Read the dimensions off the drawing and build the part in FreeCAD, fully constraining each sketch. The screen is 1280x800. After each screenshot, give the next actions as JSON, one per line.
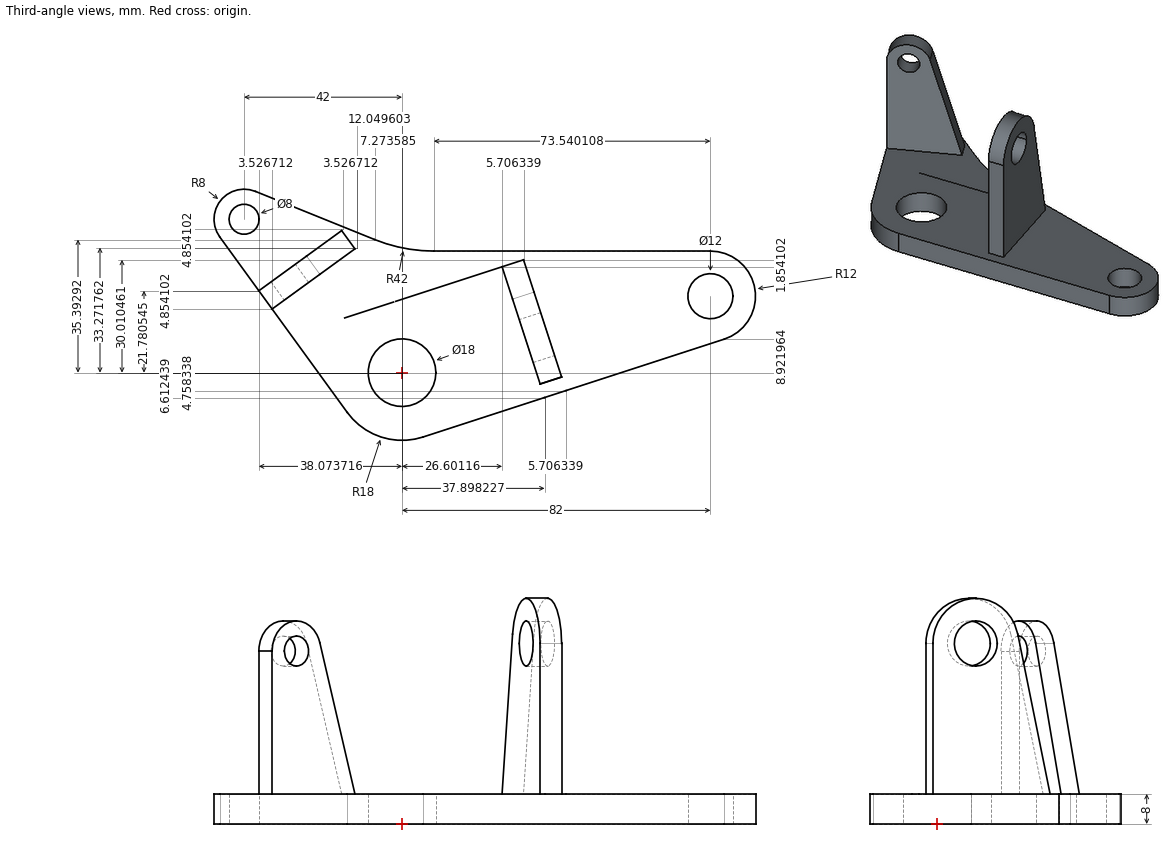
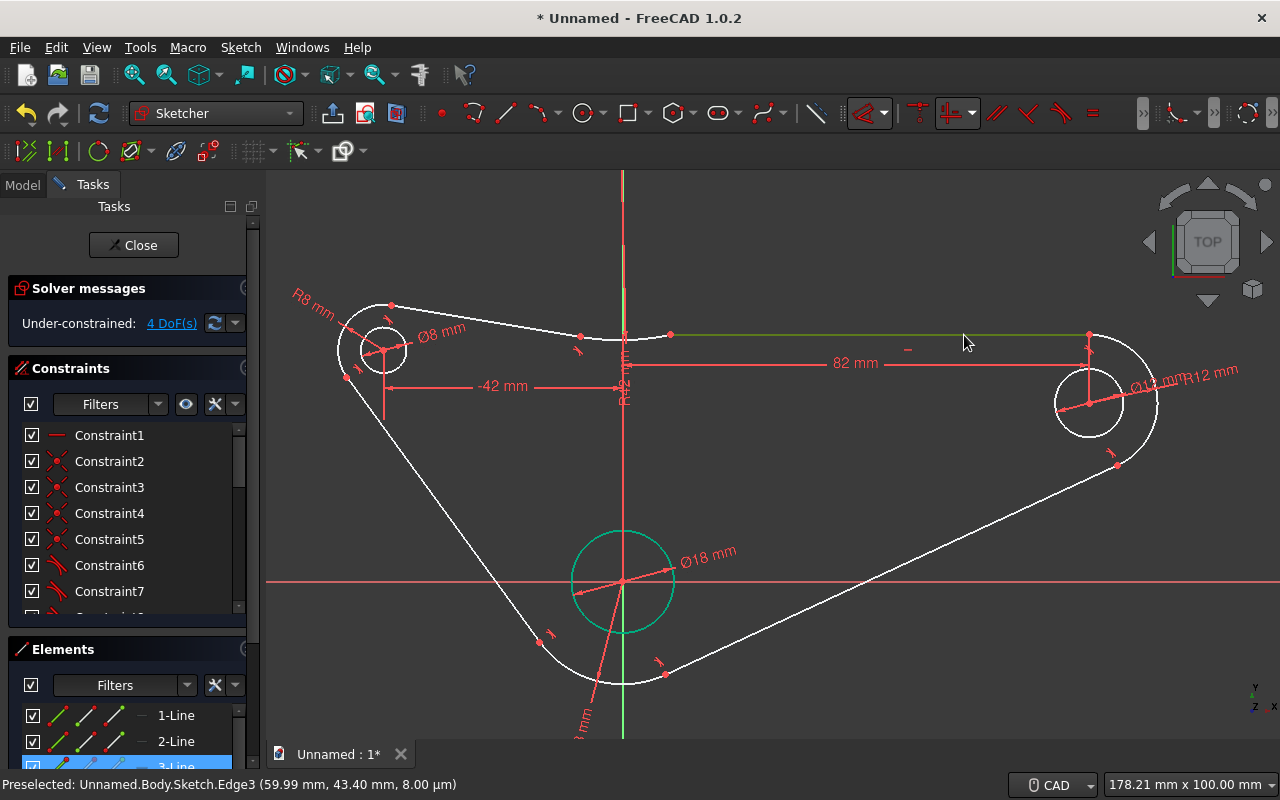
{"action": "key", "text": "l"}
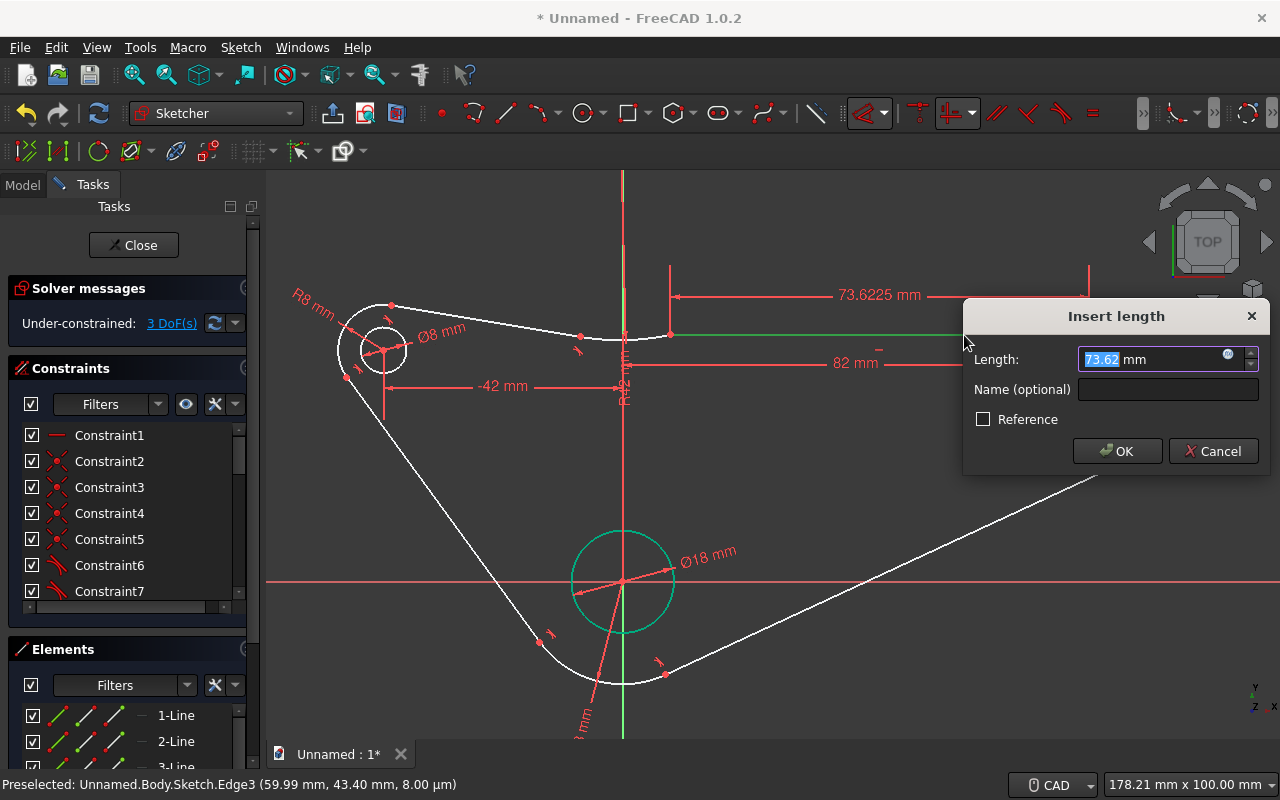
{"action": "type", "text": "73.540108"}
{"action": "key", "text": "Return"}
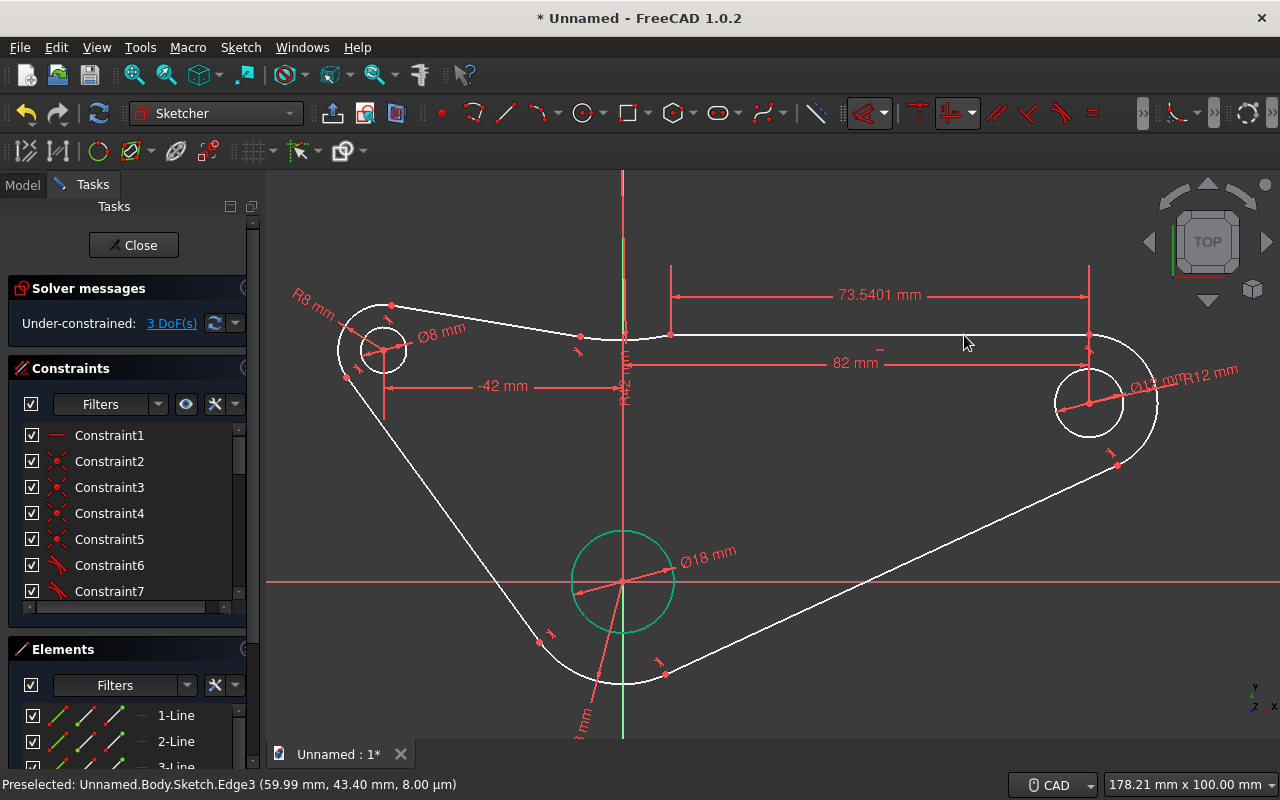
{"action": "scroll", "coordinate": [608, 376], "scroll_direction": "down", "scroll_amount": 2}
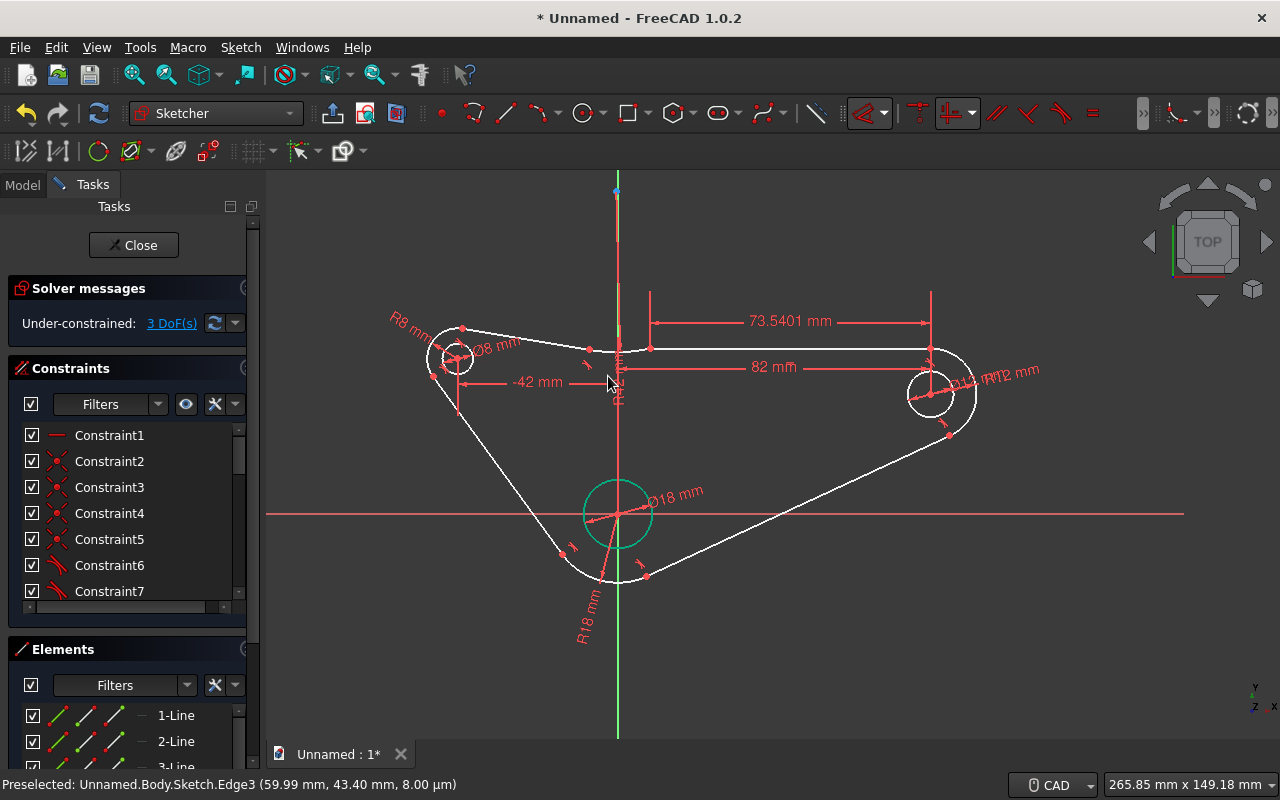
{"action": "left_click", "coordinate": [950, 436]}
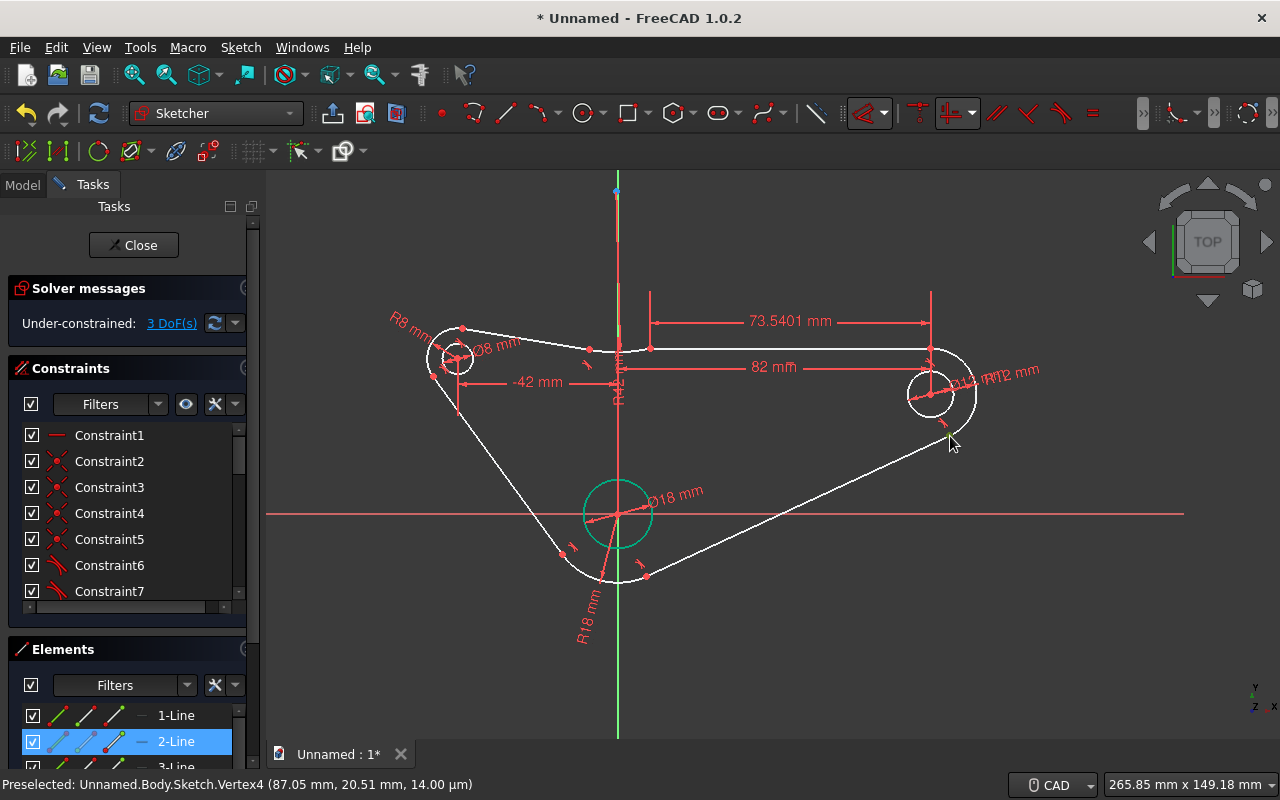
{"action": "left_click", "coordinate": [886, 114]}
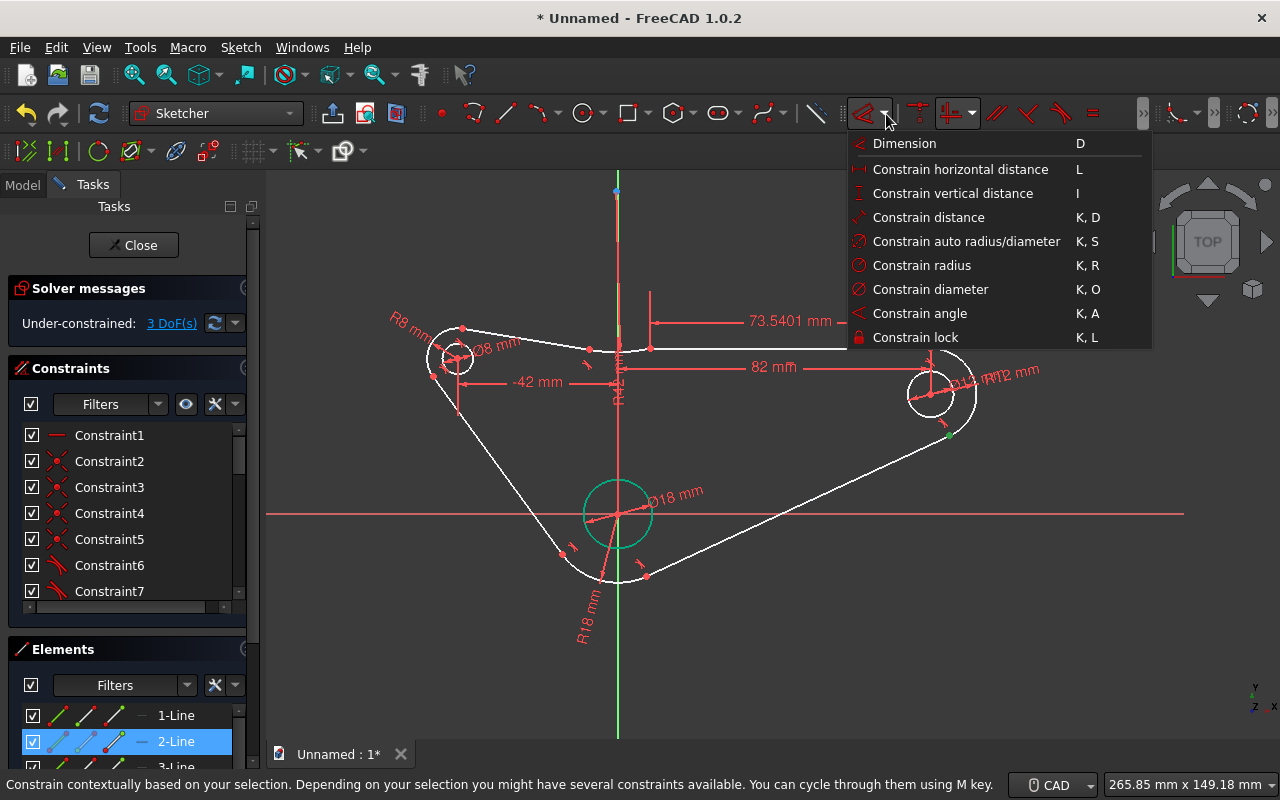
{"action": "left_click", "coordinate": [1000, 193]}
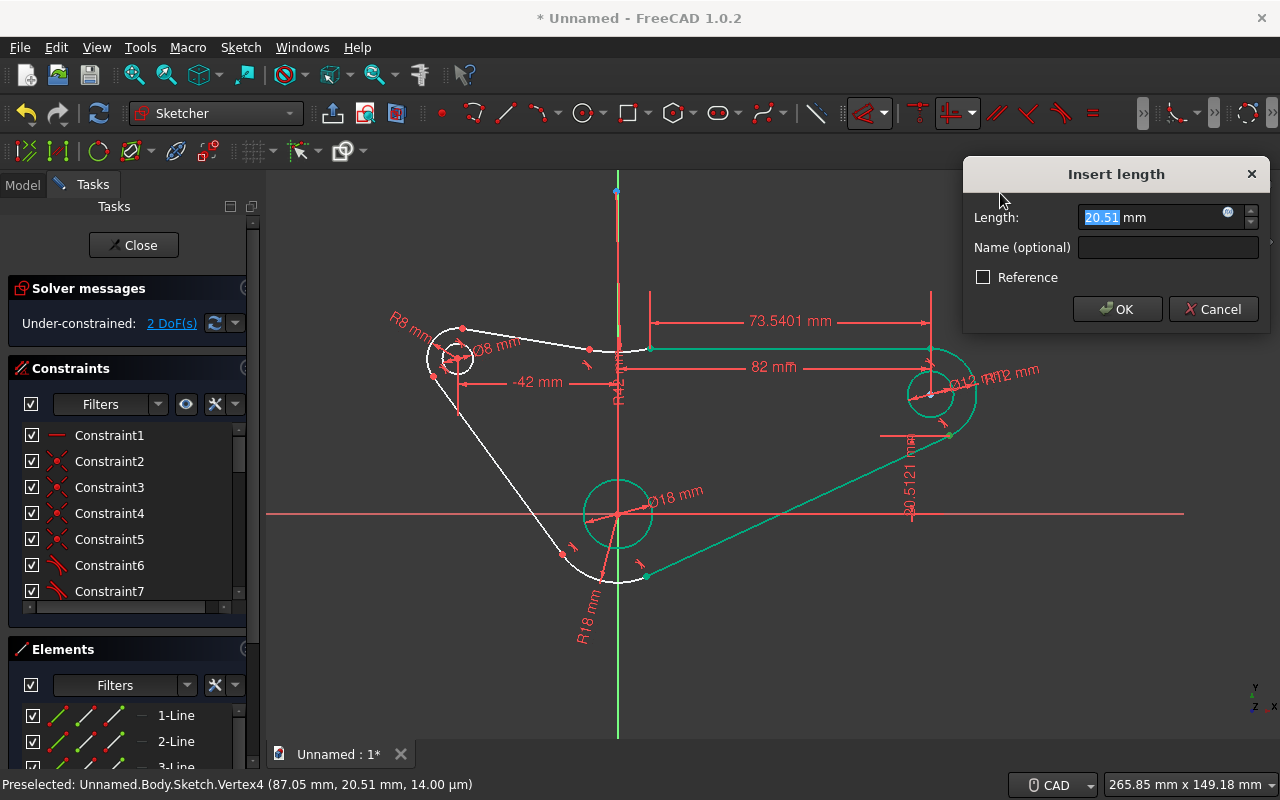
{"action": "type", "text": "8.921964"}
{"action": "key", "text": "Return"}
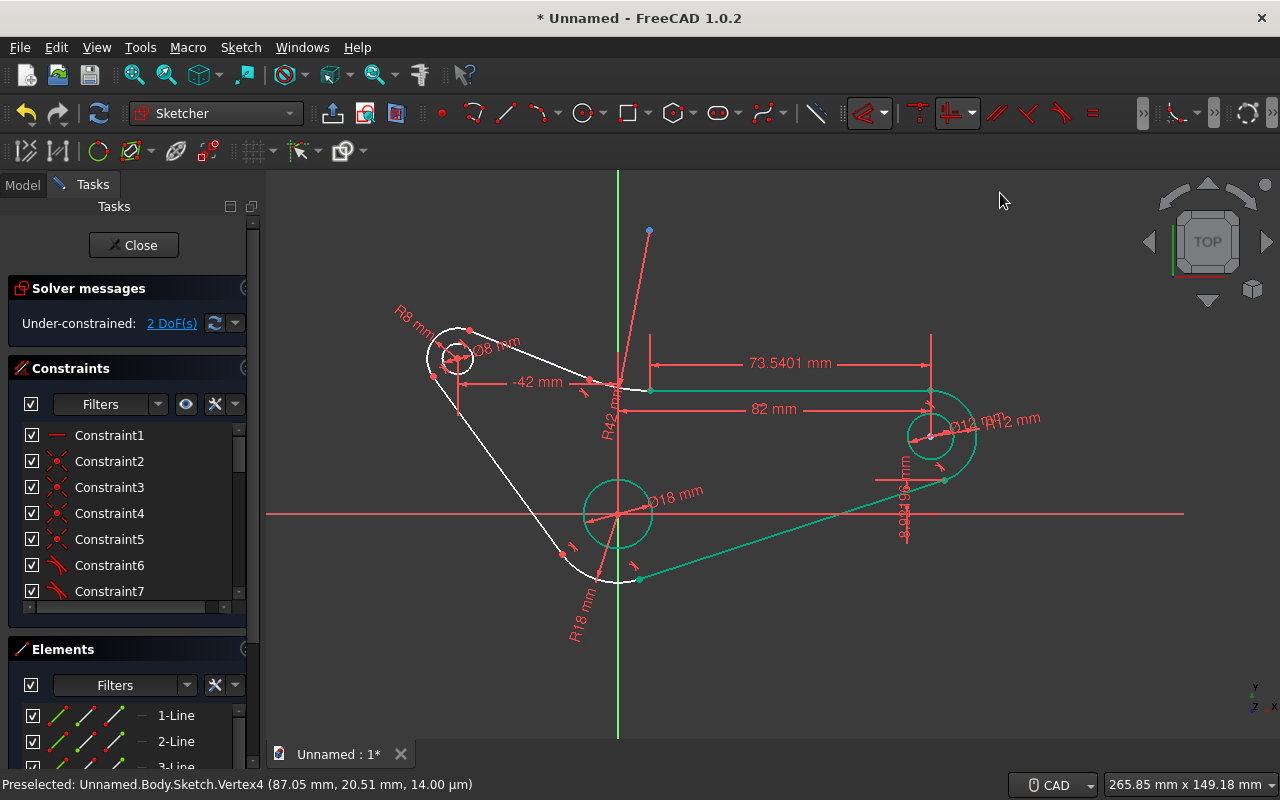
{"action": "scroll", "coordinate": [590, 379], "scroll_direction": "up", "scroll_amount": 2}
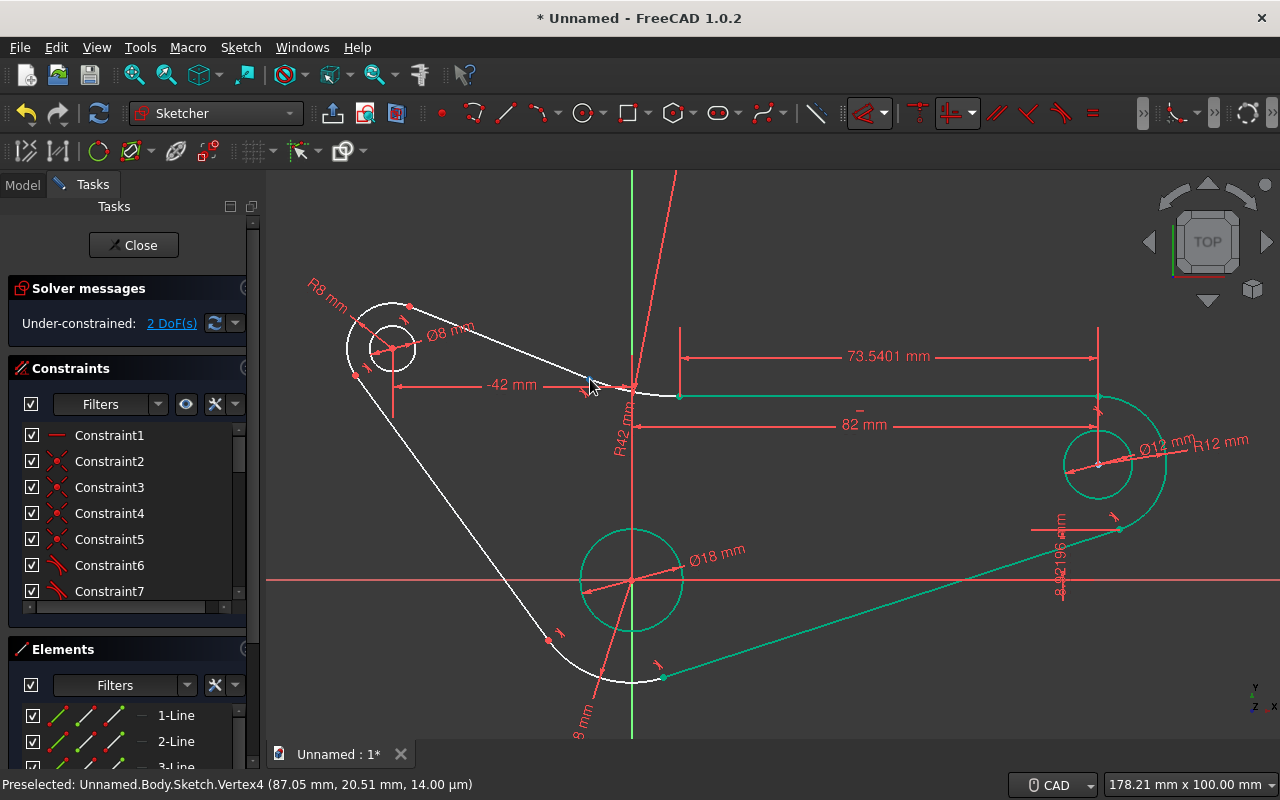
{"action": "left_click", "coordinate": [590, 379]}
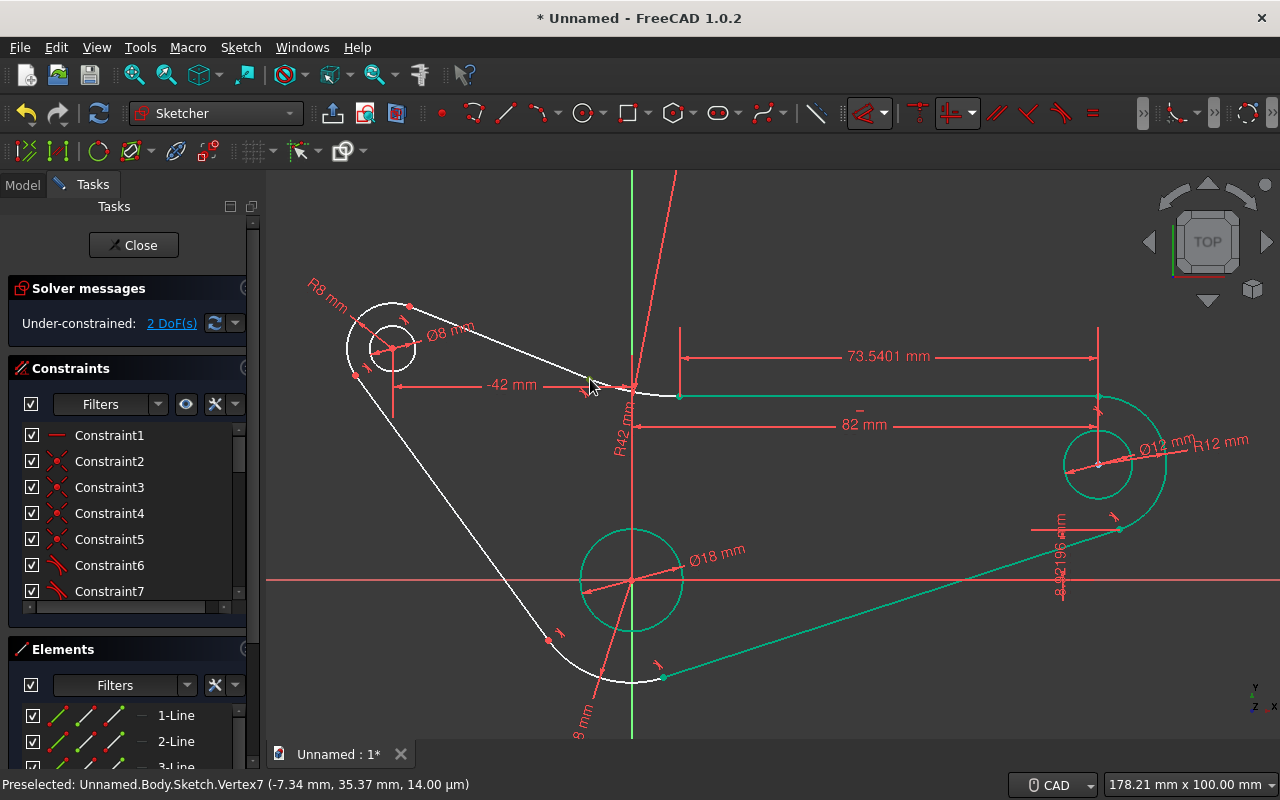
{"action": "left_click", "coordinate": [886, 114]}